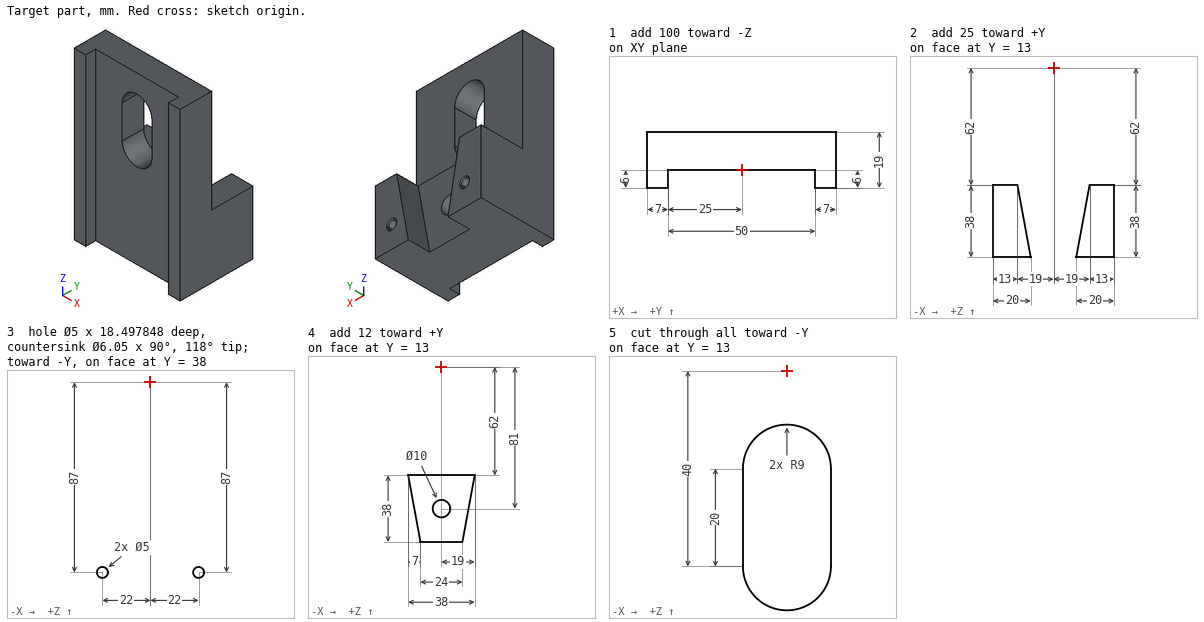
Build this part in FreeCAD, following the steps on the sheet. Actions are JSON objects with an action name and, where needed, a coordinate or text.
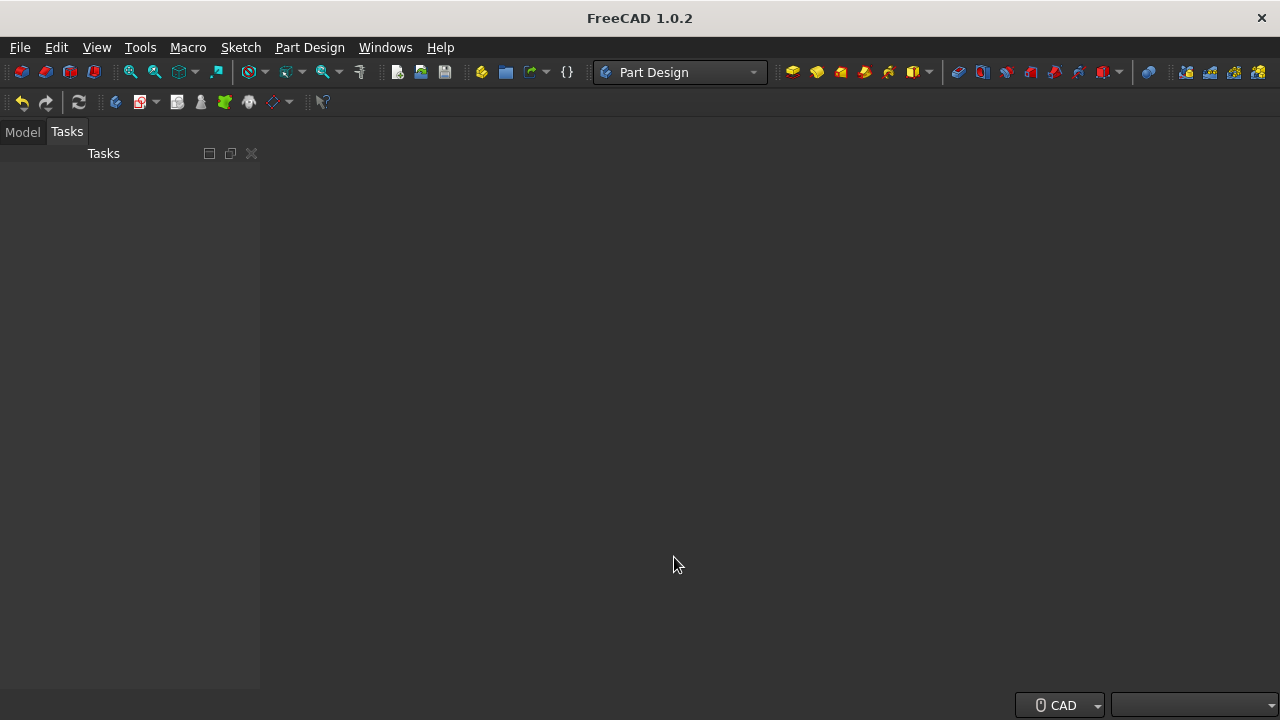
{"action": "key", "text": "ctrl+n"}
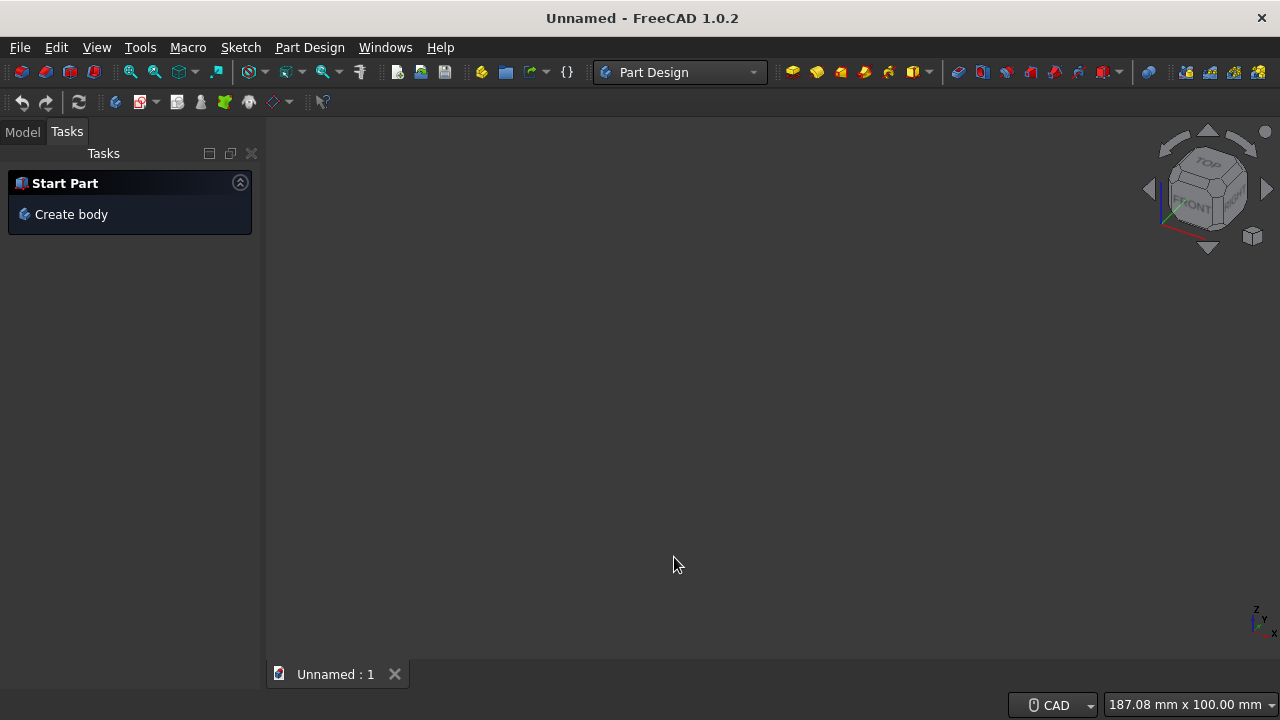
{"action": "left_click", "coordinate": [140, 102]}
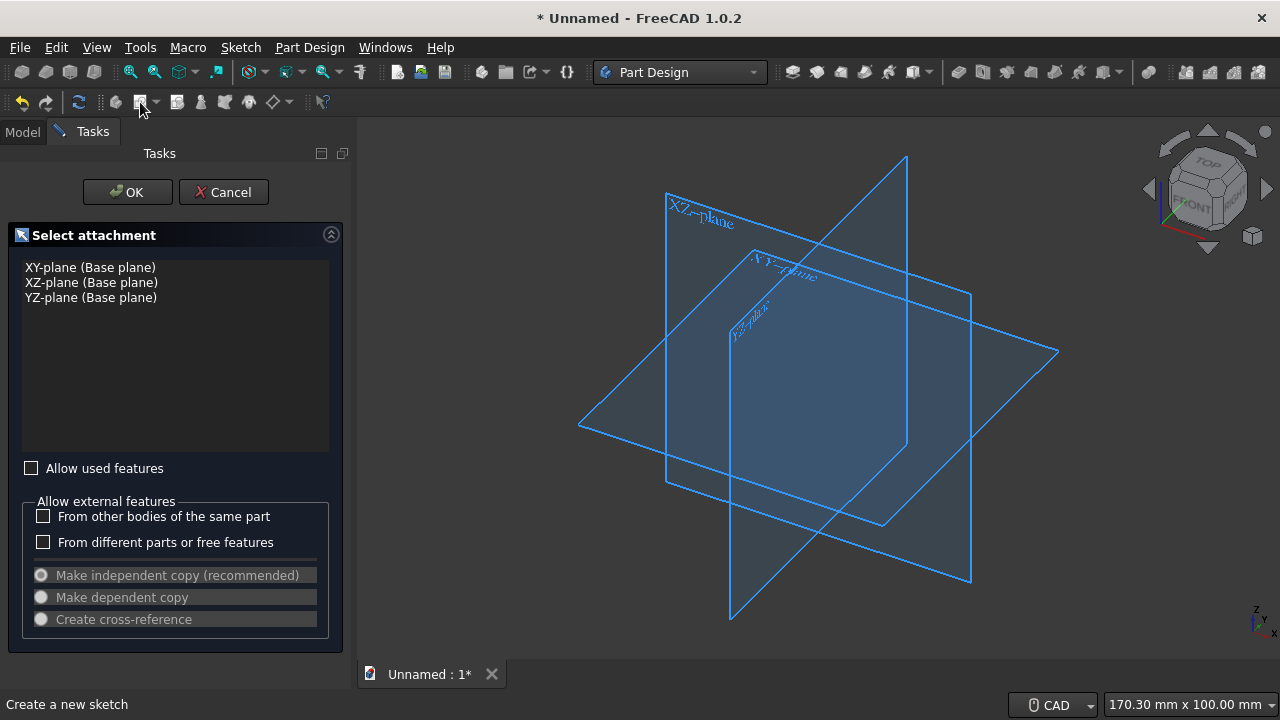
{"action": "left_click", "coordinate": [82, 268]}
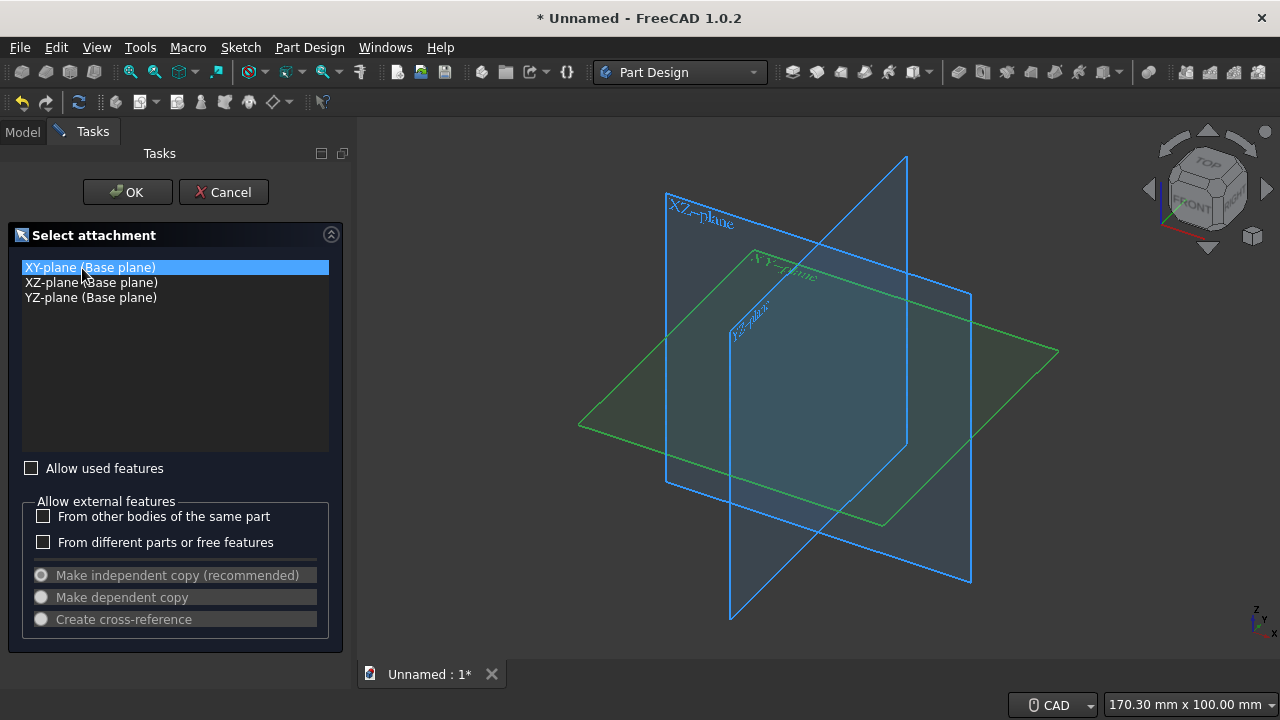
{"action": "left_click", "coordinate": [128, 192]}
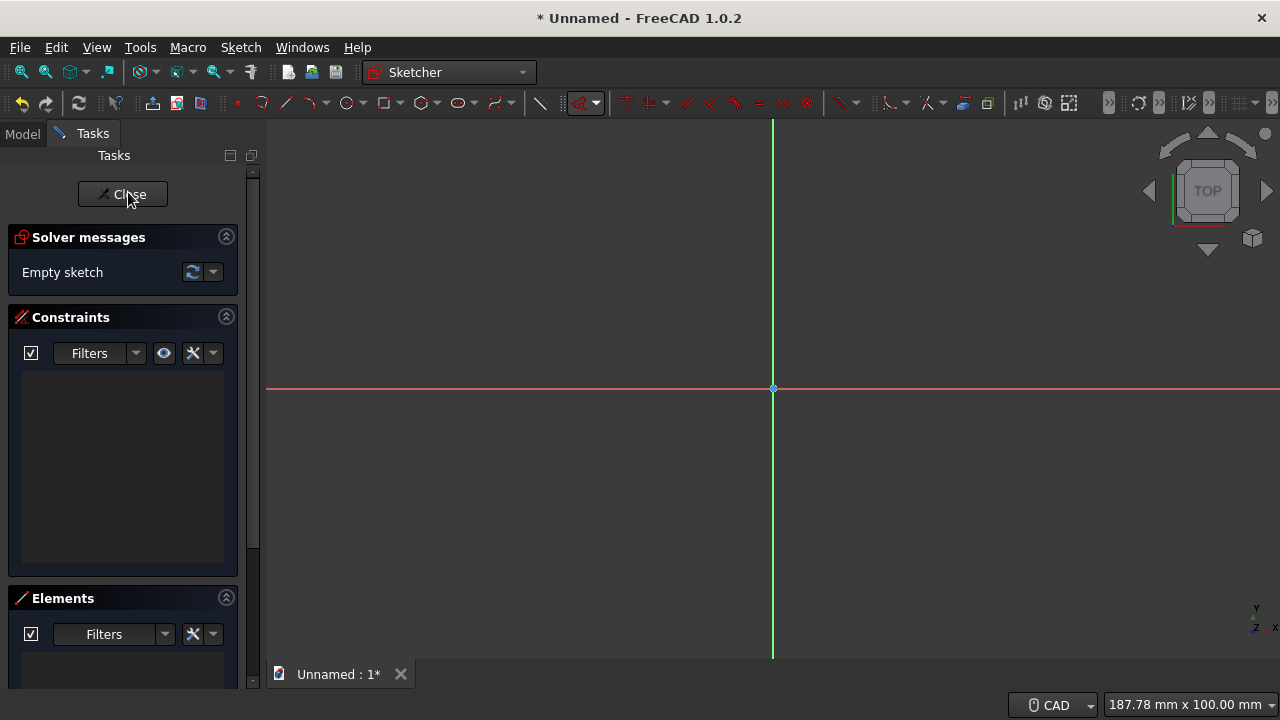
{"action": "scroll", "coordinate": [856, 347], "scroll_direction": "up", "scroll_amount": 3}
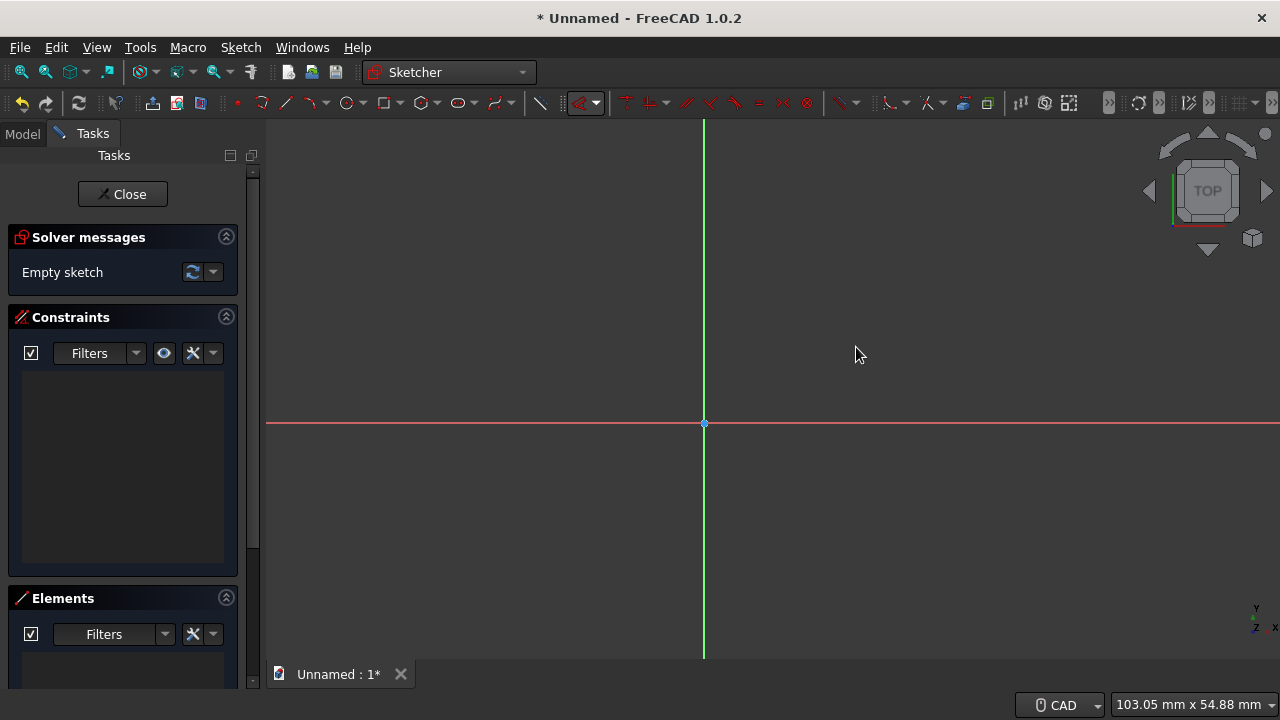
{"action": "key", "text": "g m"}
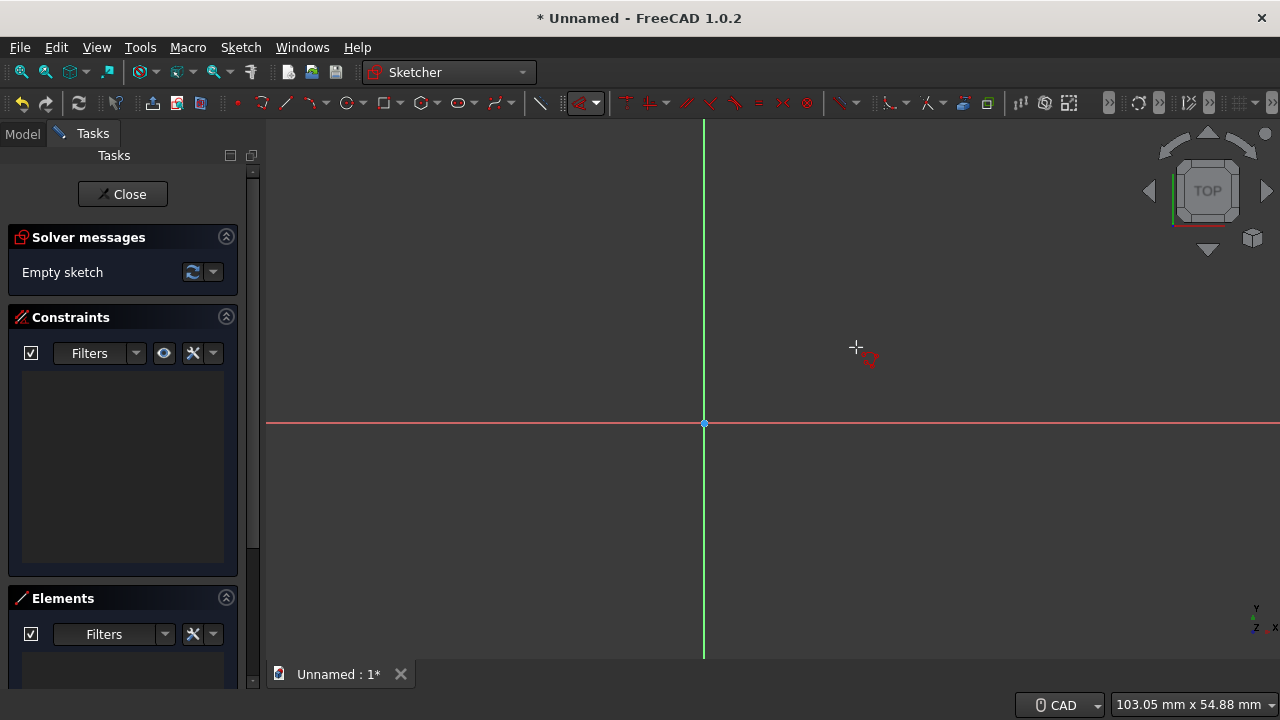
{"action": "left_click", "coordinate": [458, 423]}
{"action": "left_click", "coordinate": [950, 414]}
{"action": "left_click", "coordinate": [950, 482]}
{"action": "left_click", "coordinate": [1019, 482]}
{"action": "left_click", "coordinate": [1019, 295]}
{"action": "left_click", "coordinate": [389, 295]}
{"action": "left_click", "coordinate": [389, 482]}
{"action": "left_click", "coordinate": [458, 482]}
{"action": "left_click", "coordinate": [458, 423]}
{"action": "key", "text": "Escape"}
{"action": "key", "text": "Escape"}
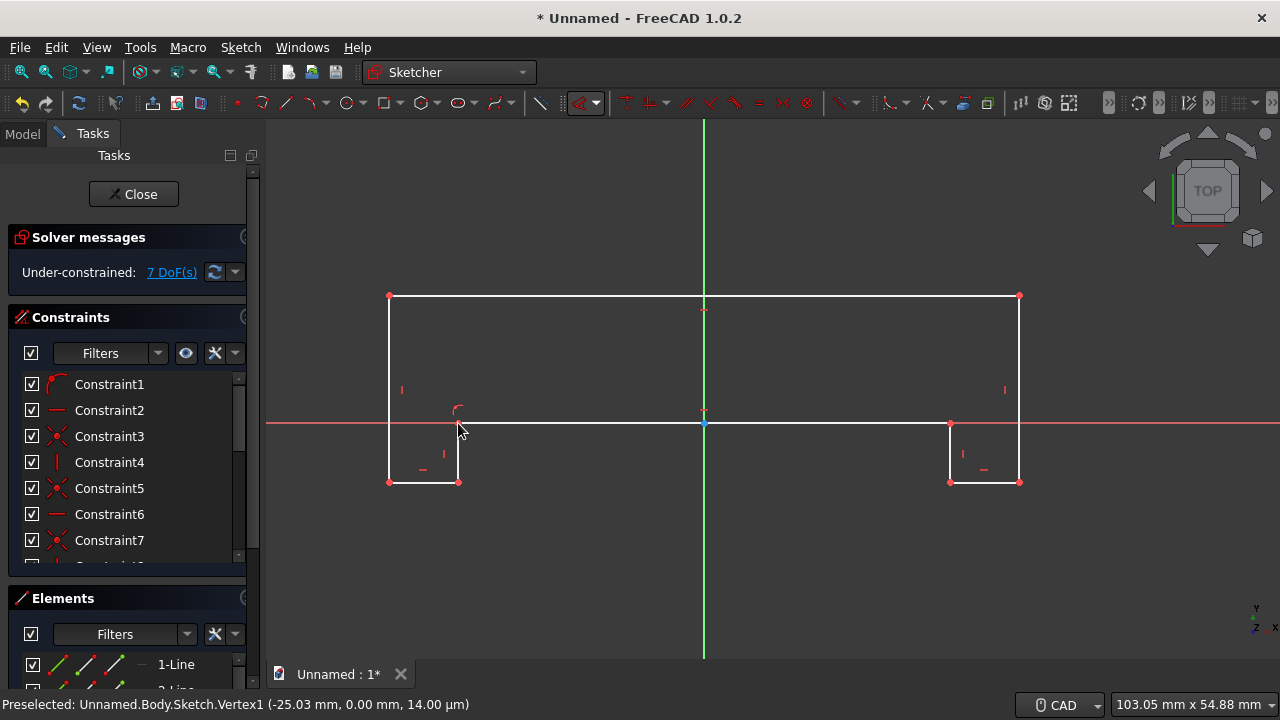
{"action": "key", "text": "d"}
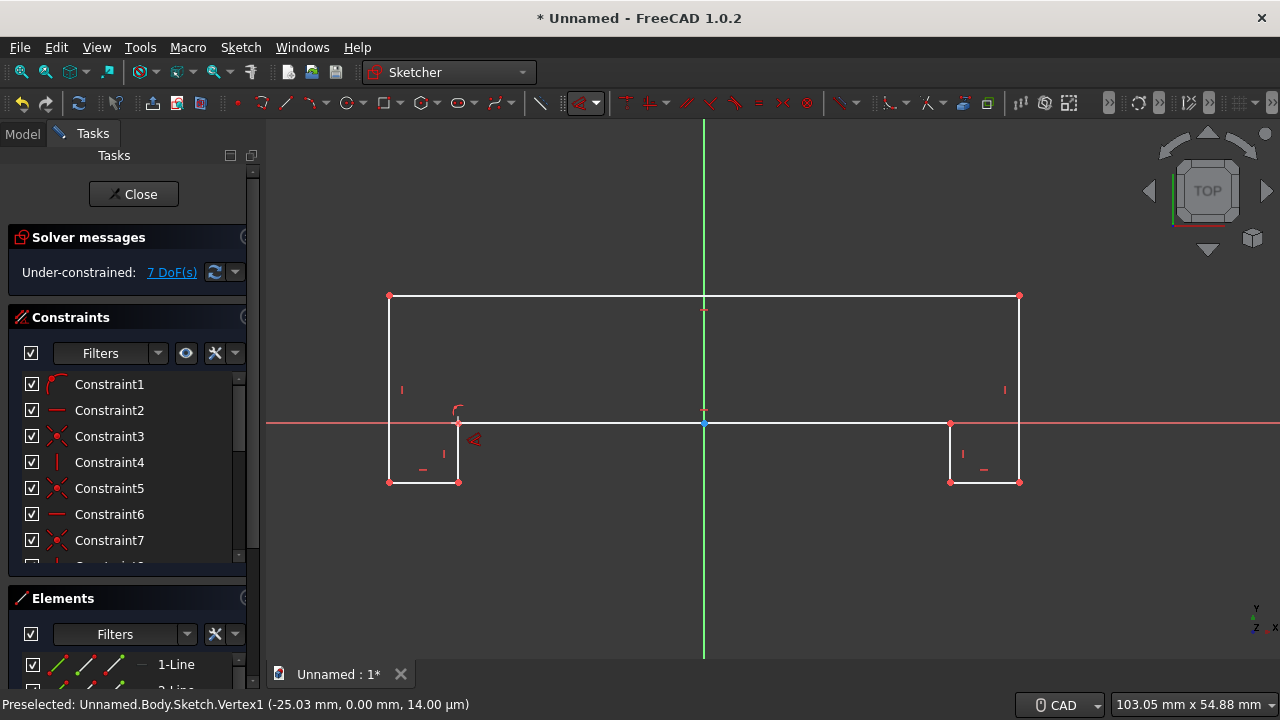
{"action": "left_click", "coordinate": [950, 441]}
{"action": "left_click", "coordinate": [984, 453]}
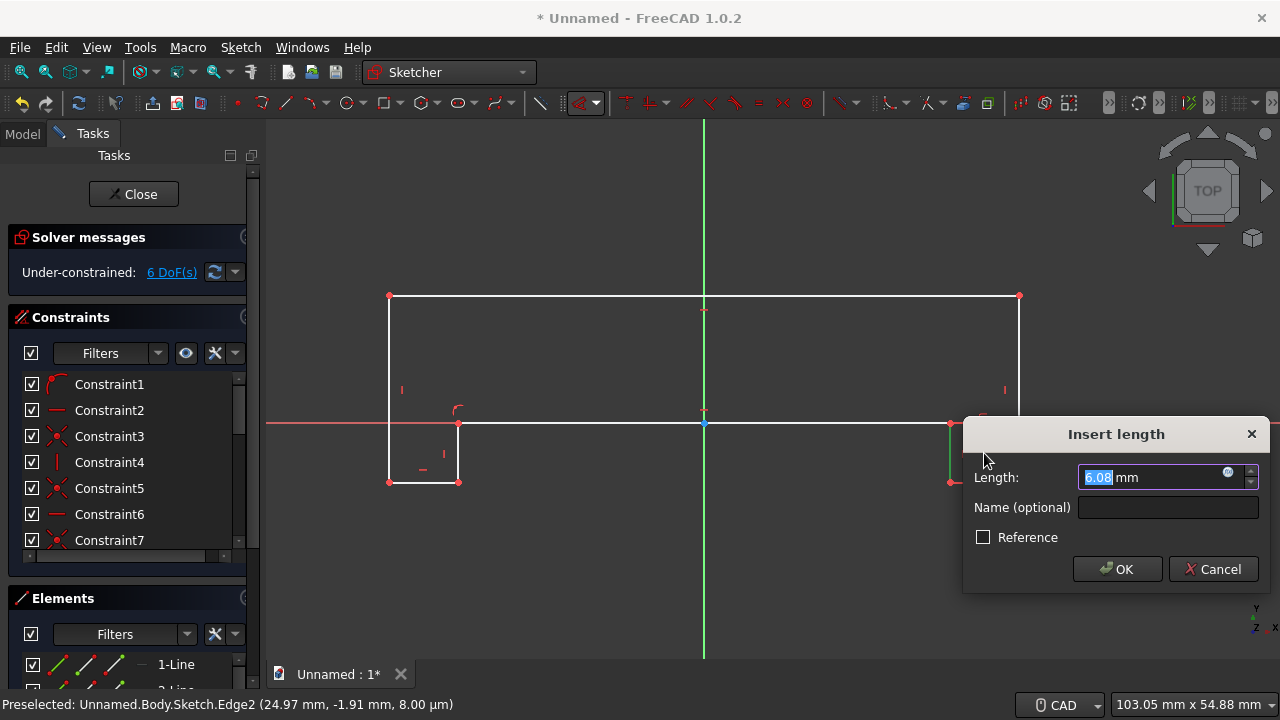
{"action": "type", "text": "6"}
{"action": "key", "text": "Return"}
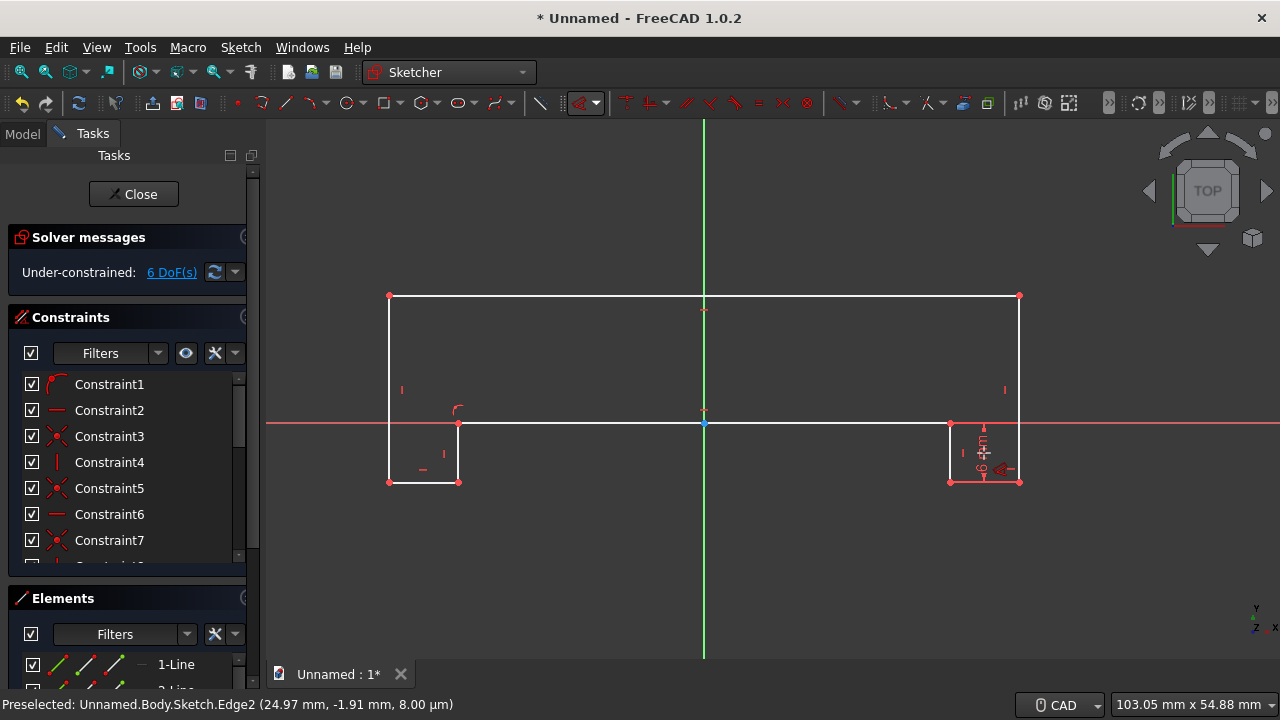
{"action": "left_click", "coordinate": [971, 482]}
{"action": "left_click", "coordinate": [984, 516]}